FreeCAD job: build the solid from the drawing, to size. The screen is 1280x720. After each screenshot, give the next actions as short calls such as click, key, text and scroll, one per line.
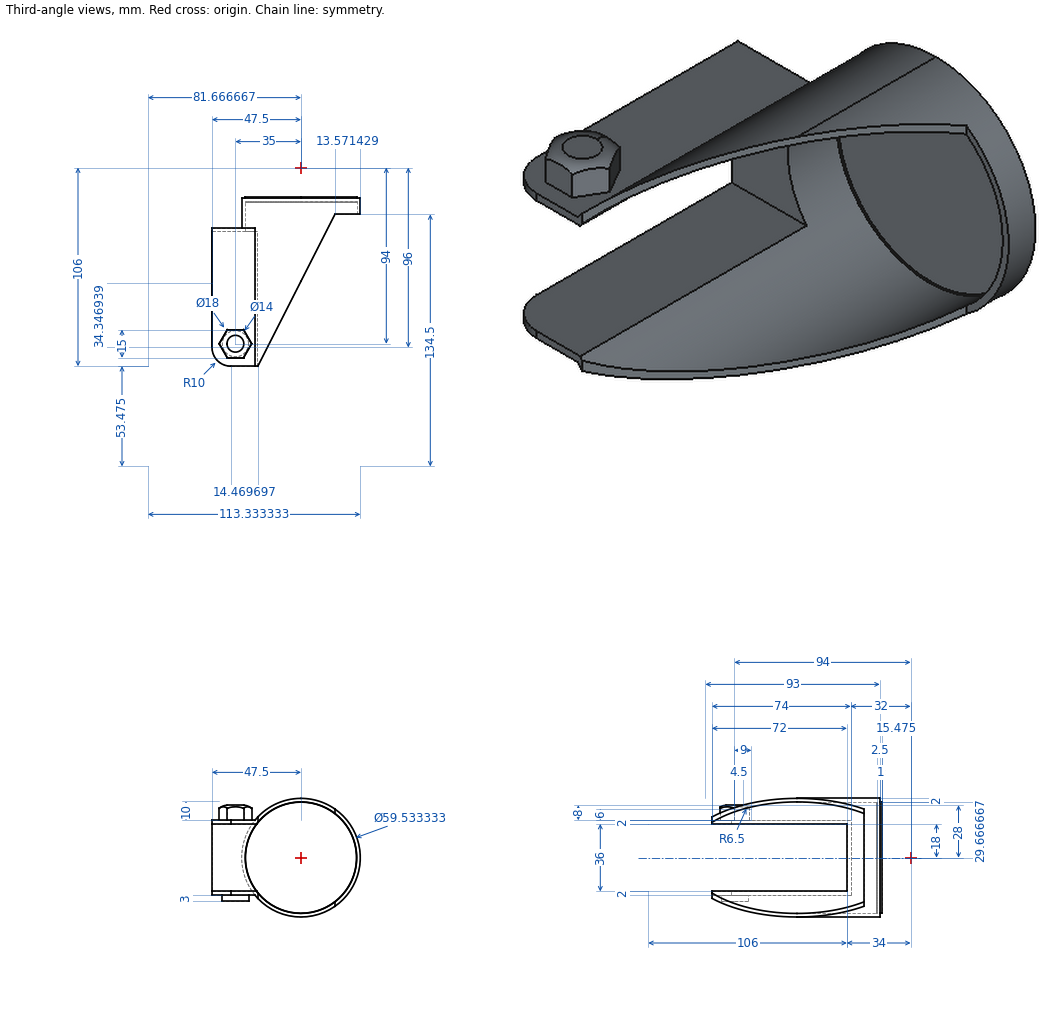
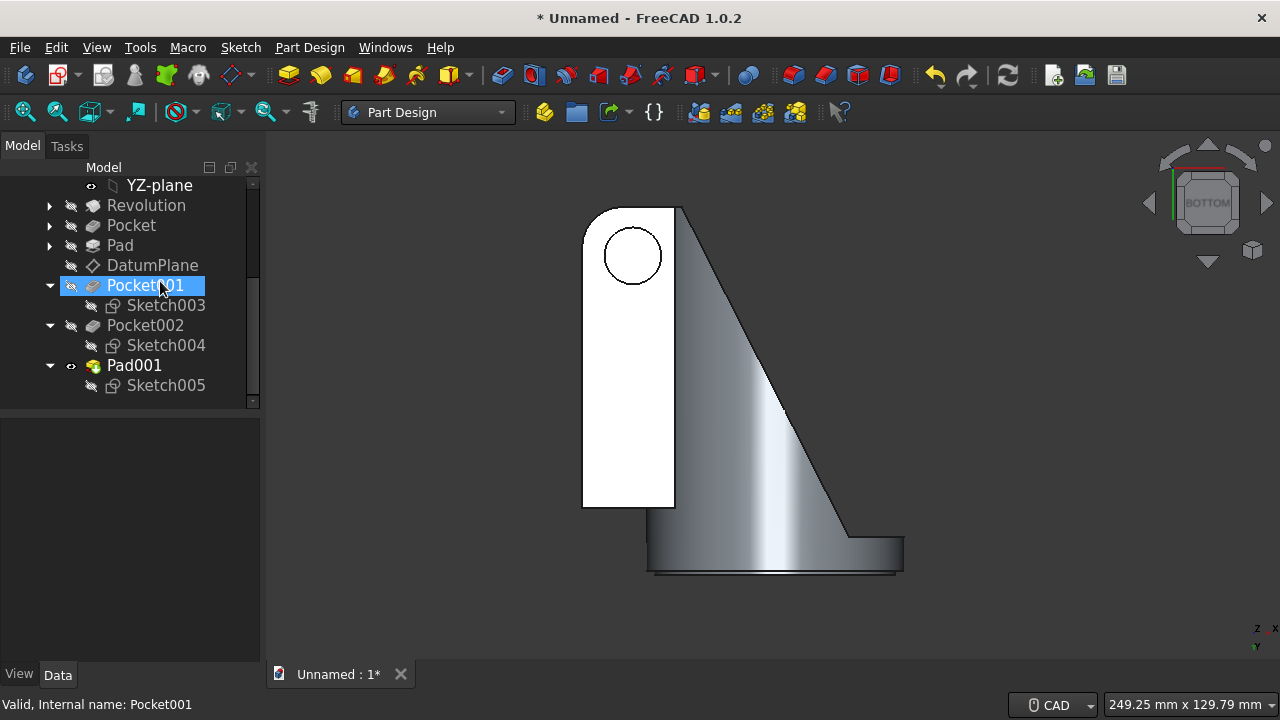
scroll(160, 281, up, 15)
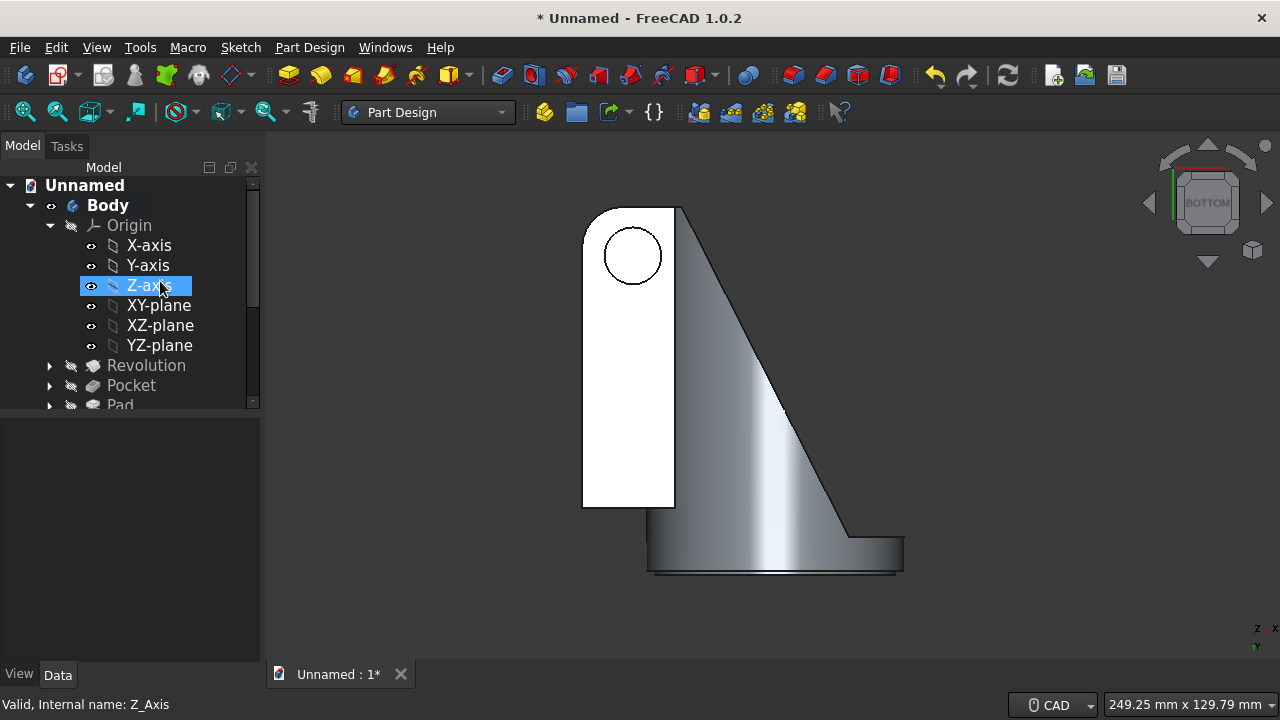
click(136, 346)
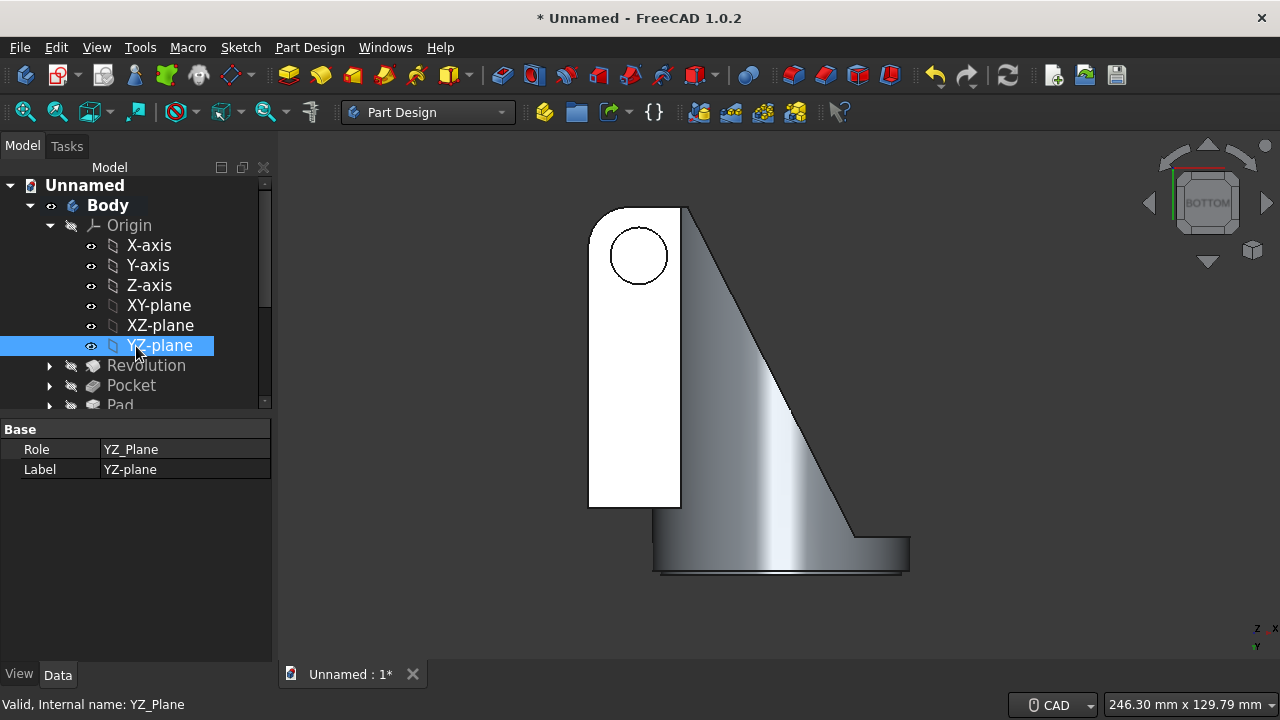
click(232, 76)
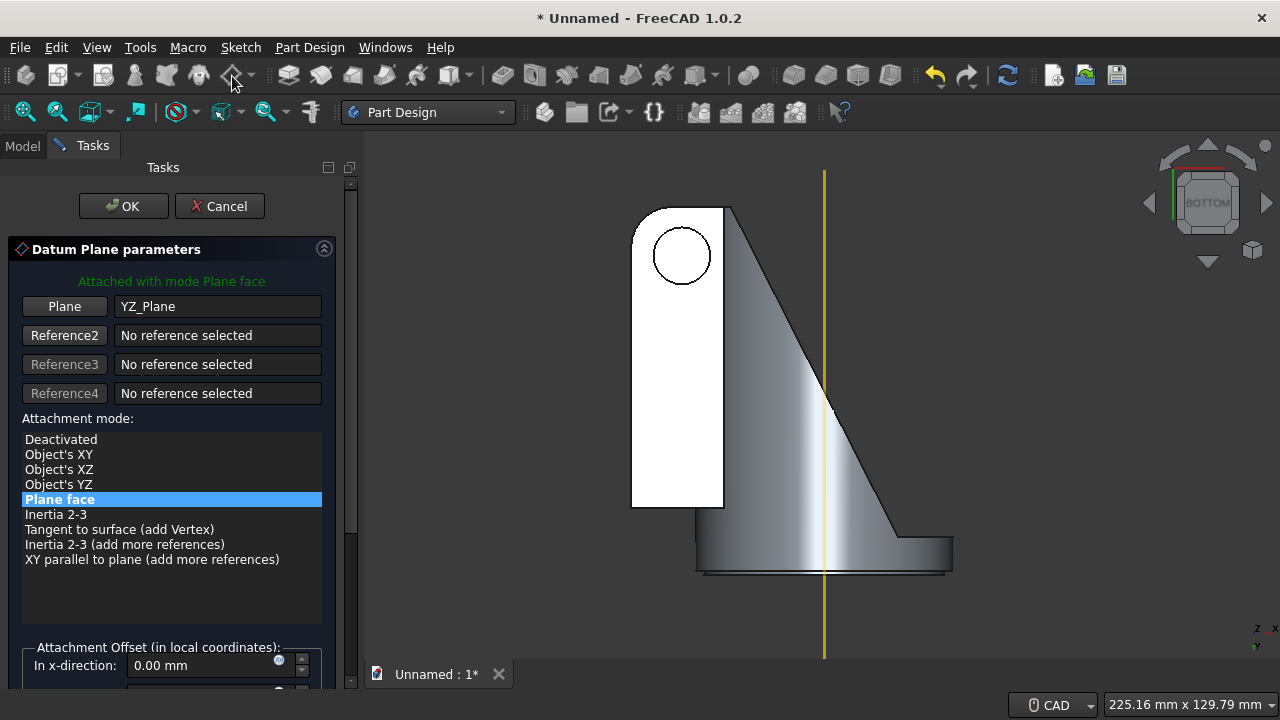
scroll(351, 432, down, 2)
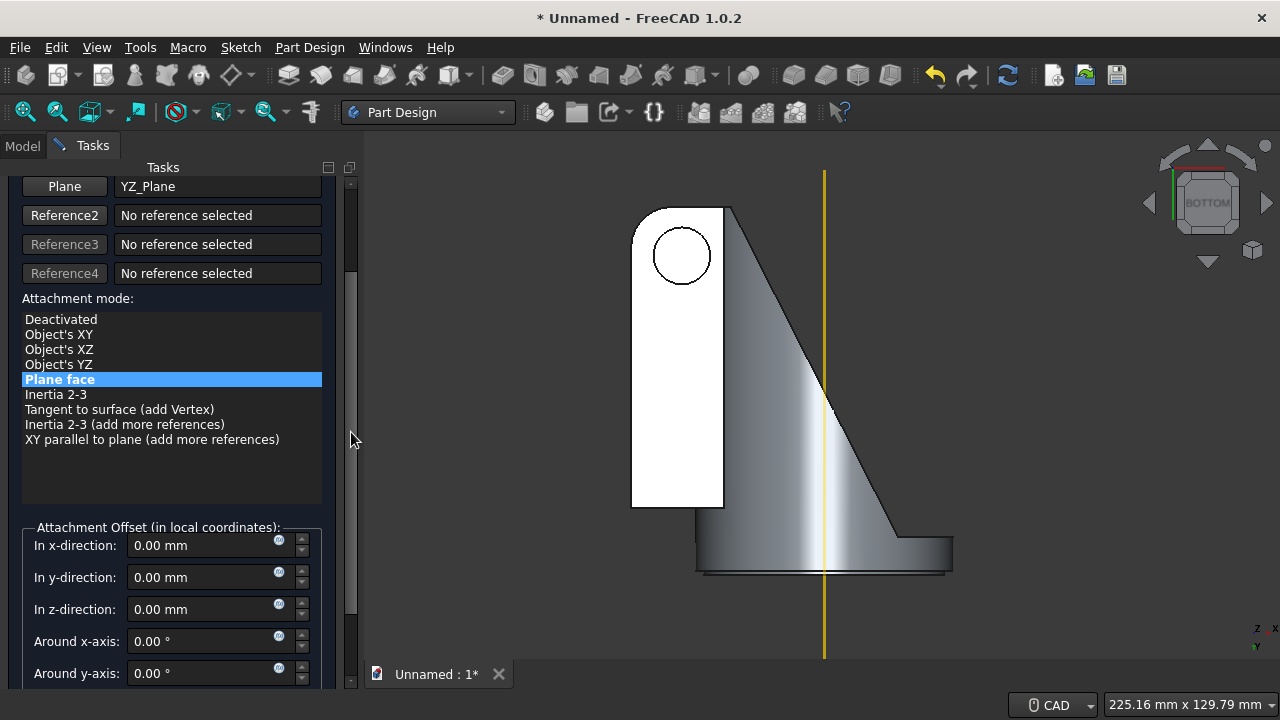
triple_click(210, 609)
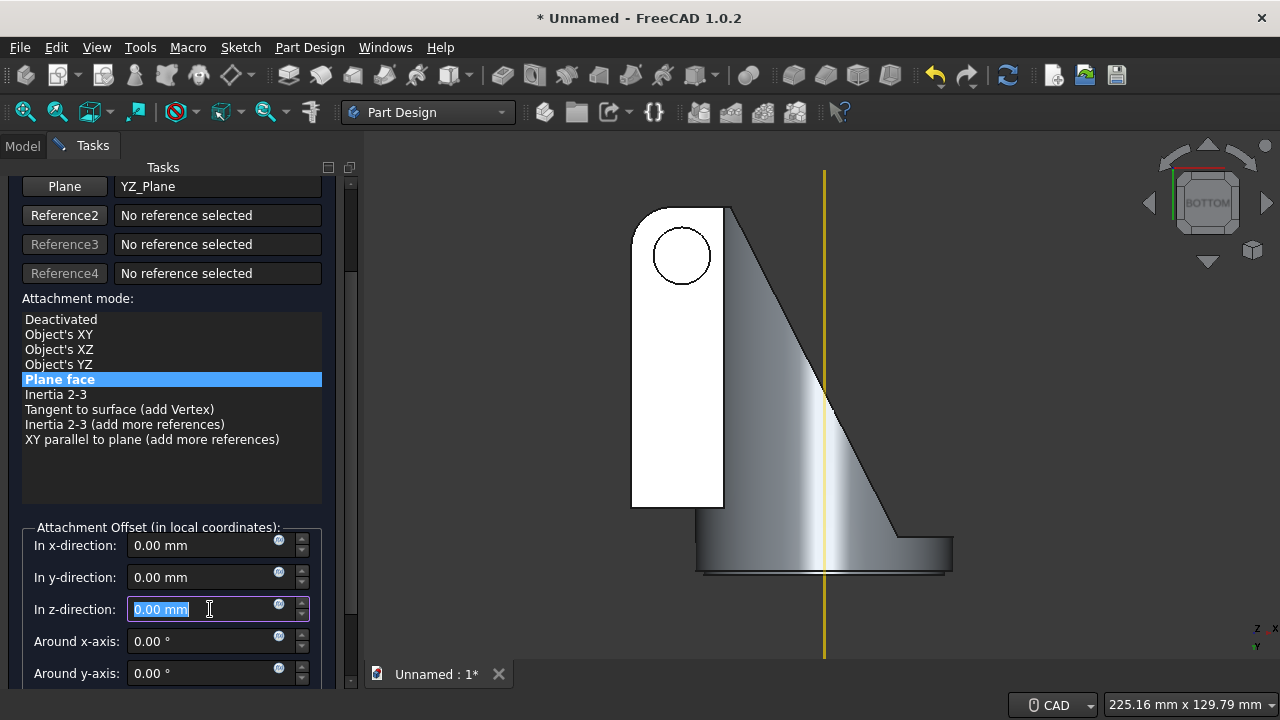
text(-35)
key(Tab)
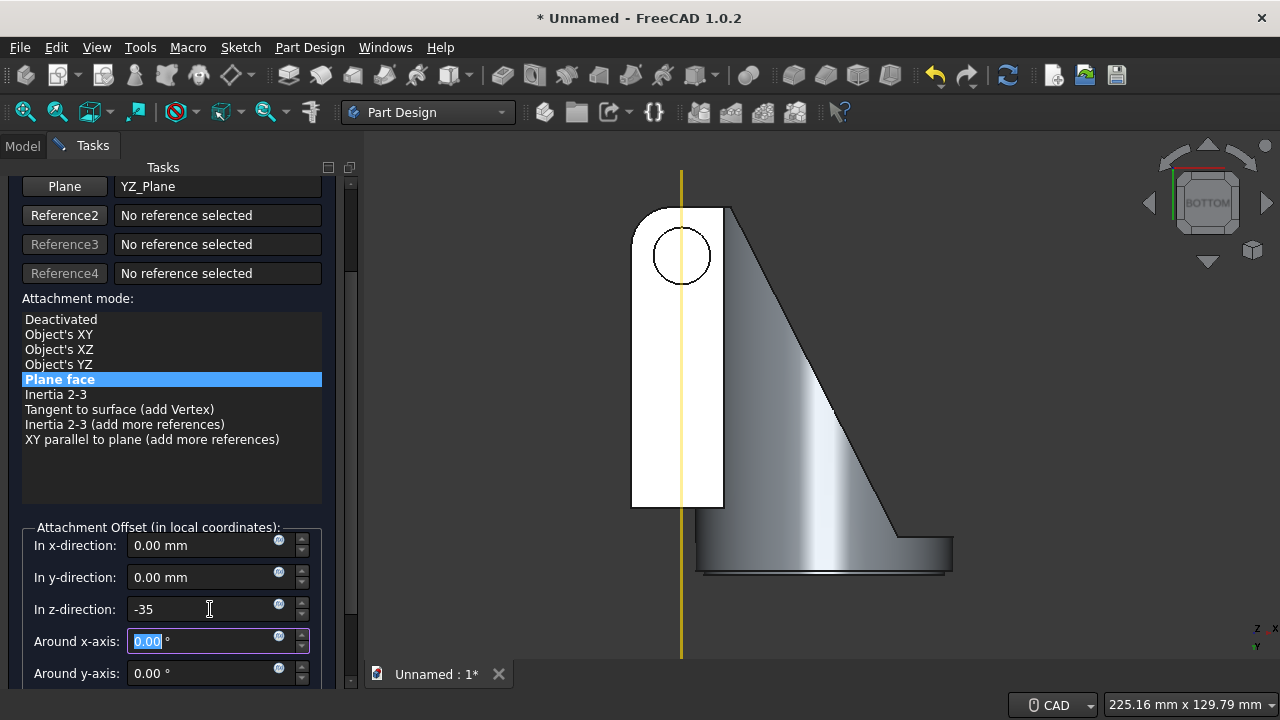
scroll(351, 432, up, 3)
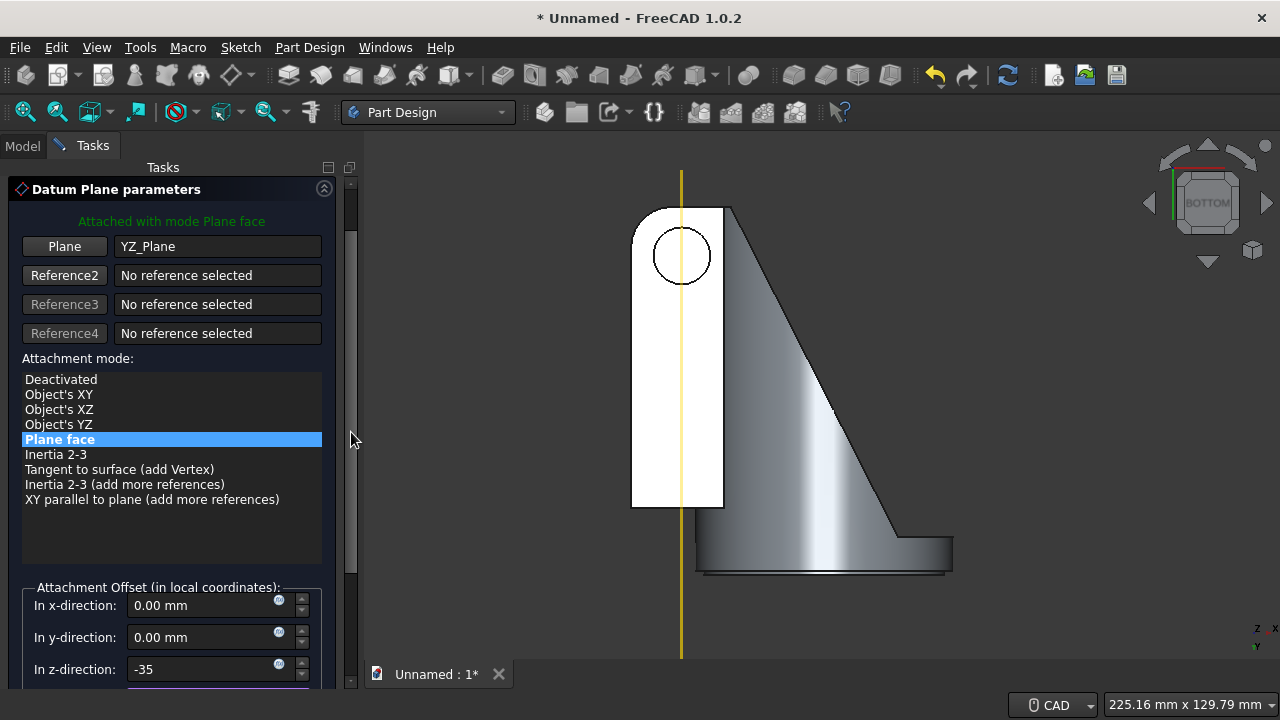
click(124, 206)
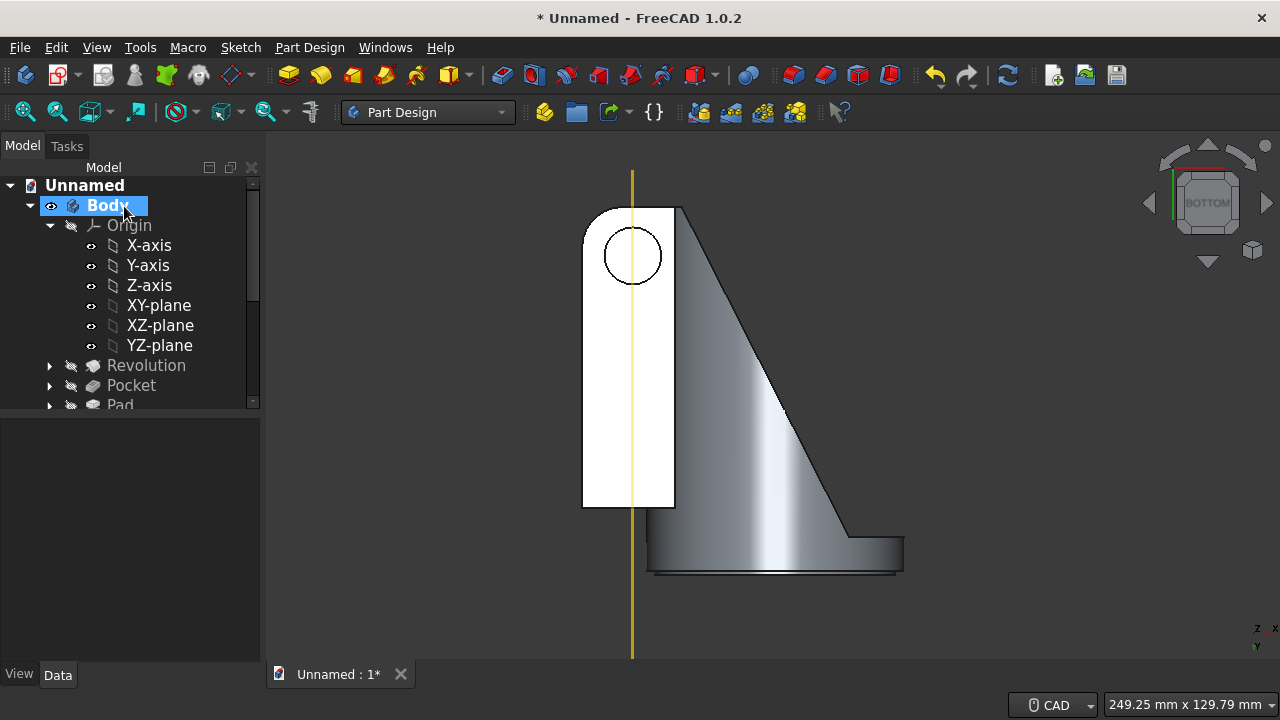
scroll(100, 301, down, 3)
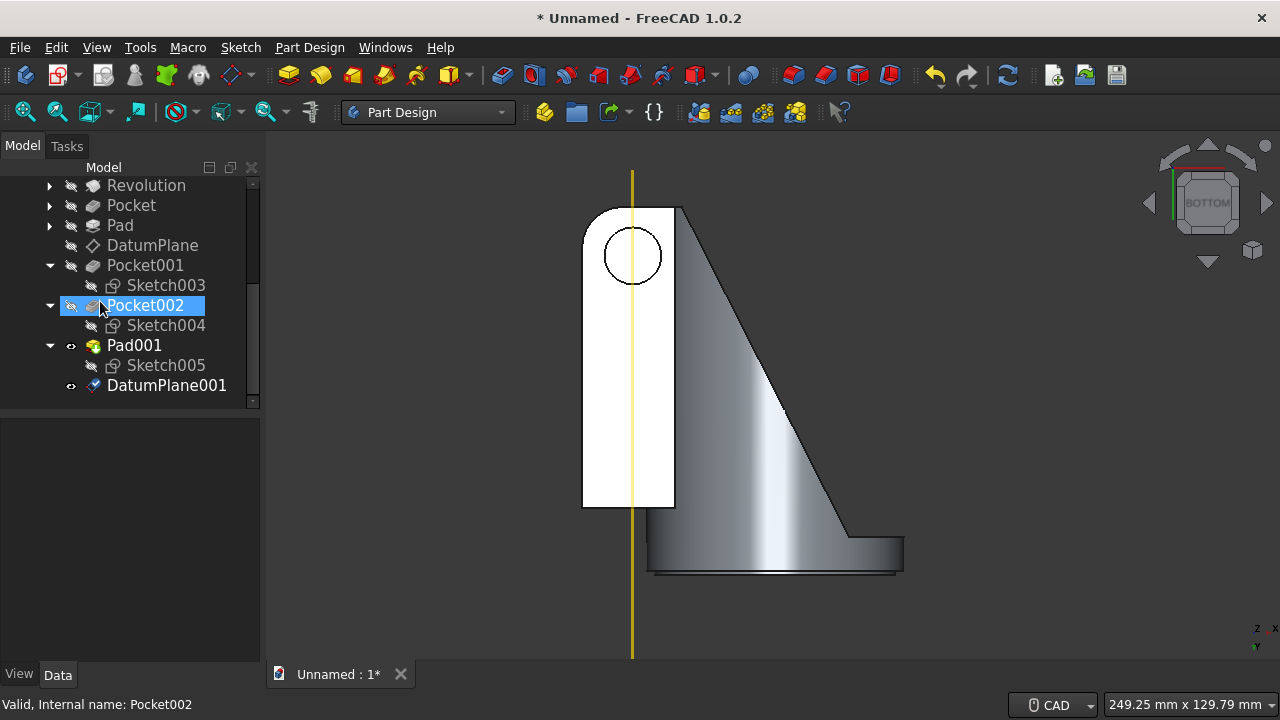
click(116, 386)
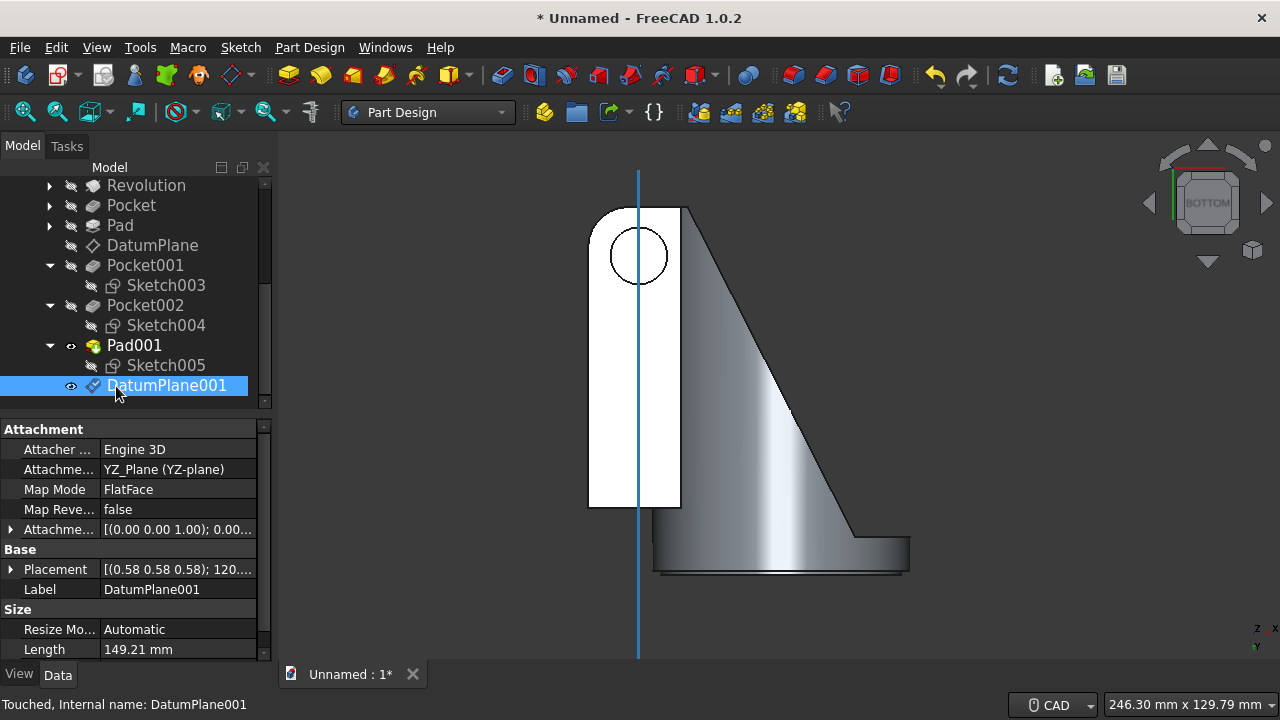
click(58, 76)